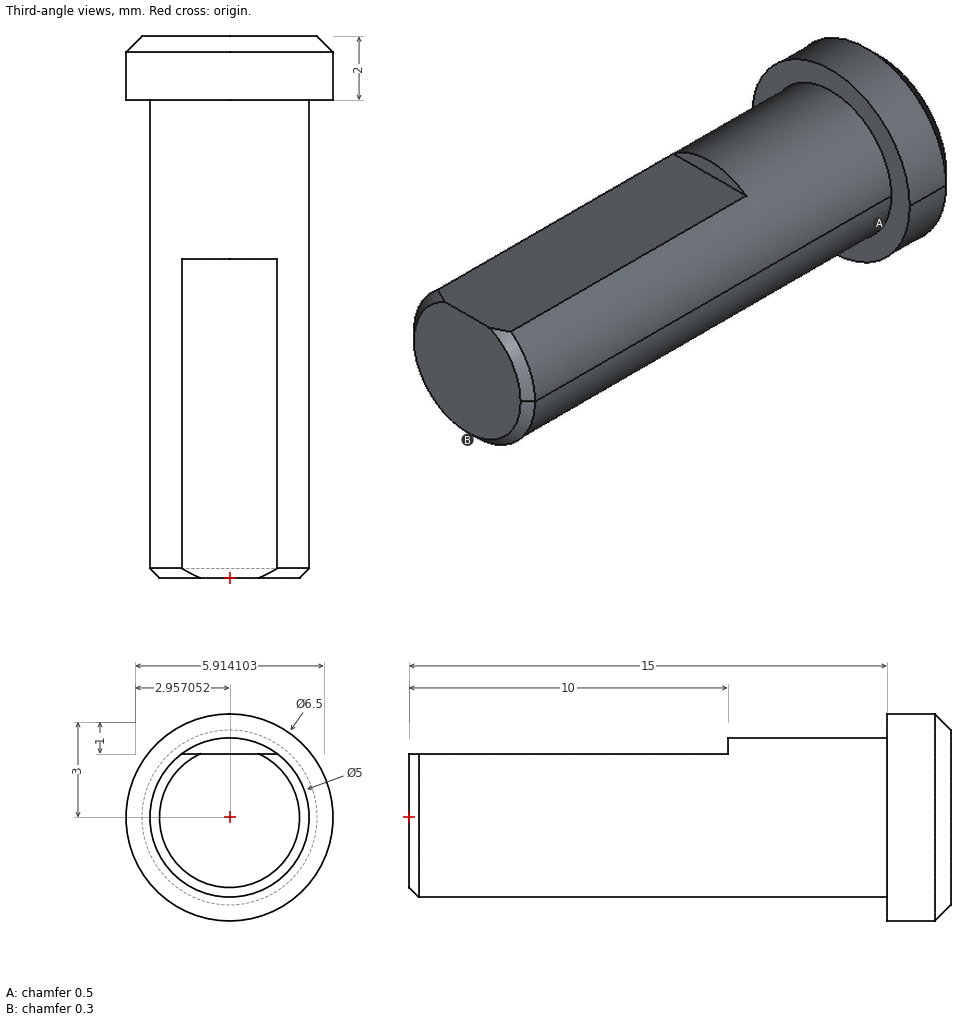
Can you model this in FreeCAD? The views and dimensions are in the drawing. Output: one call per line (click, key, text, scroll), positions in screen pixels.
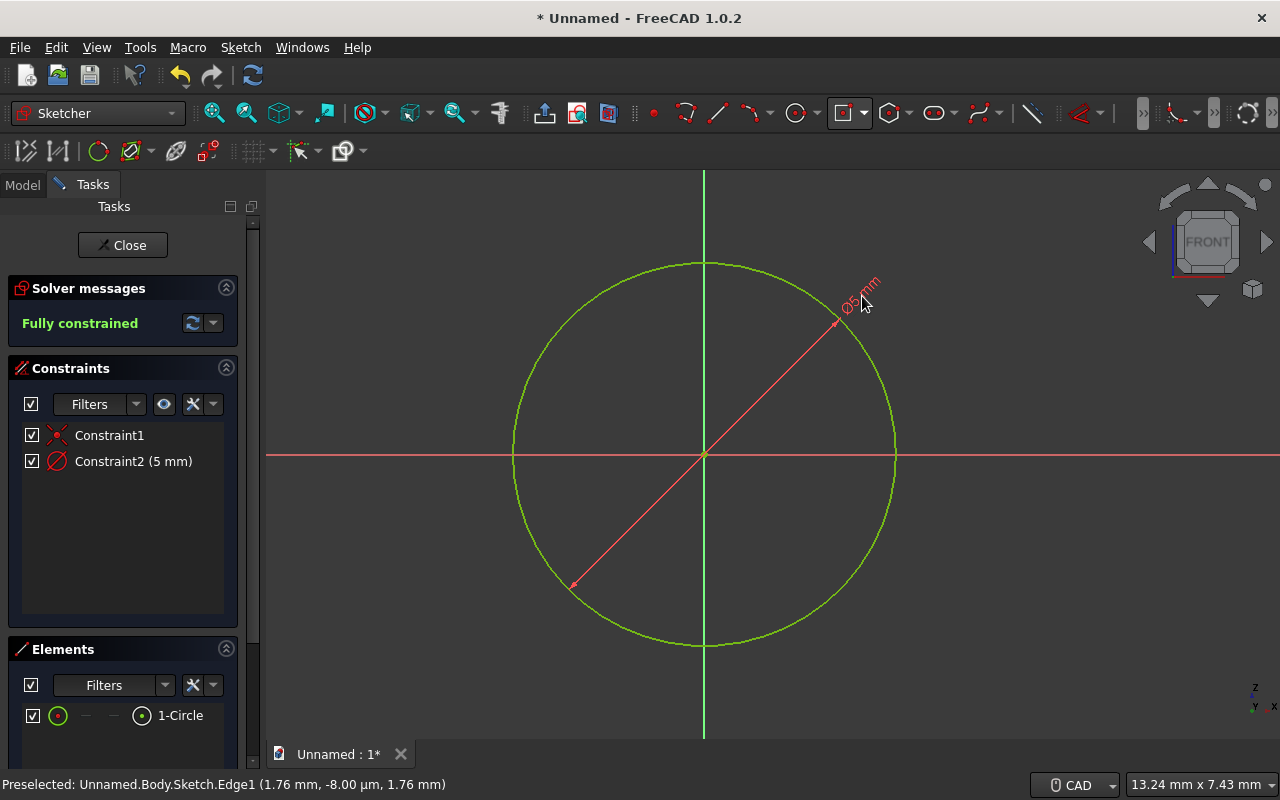
click(123, 245)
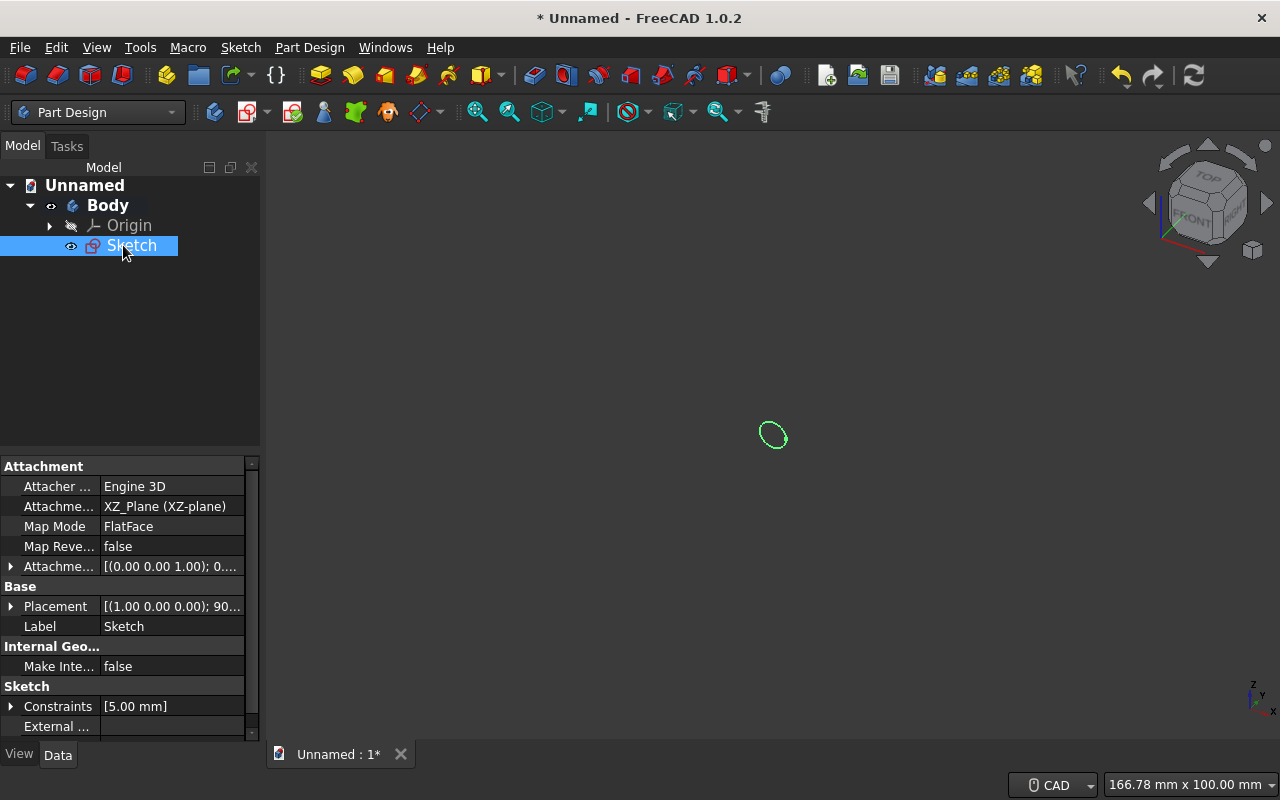
click(322, 76)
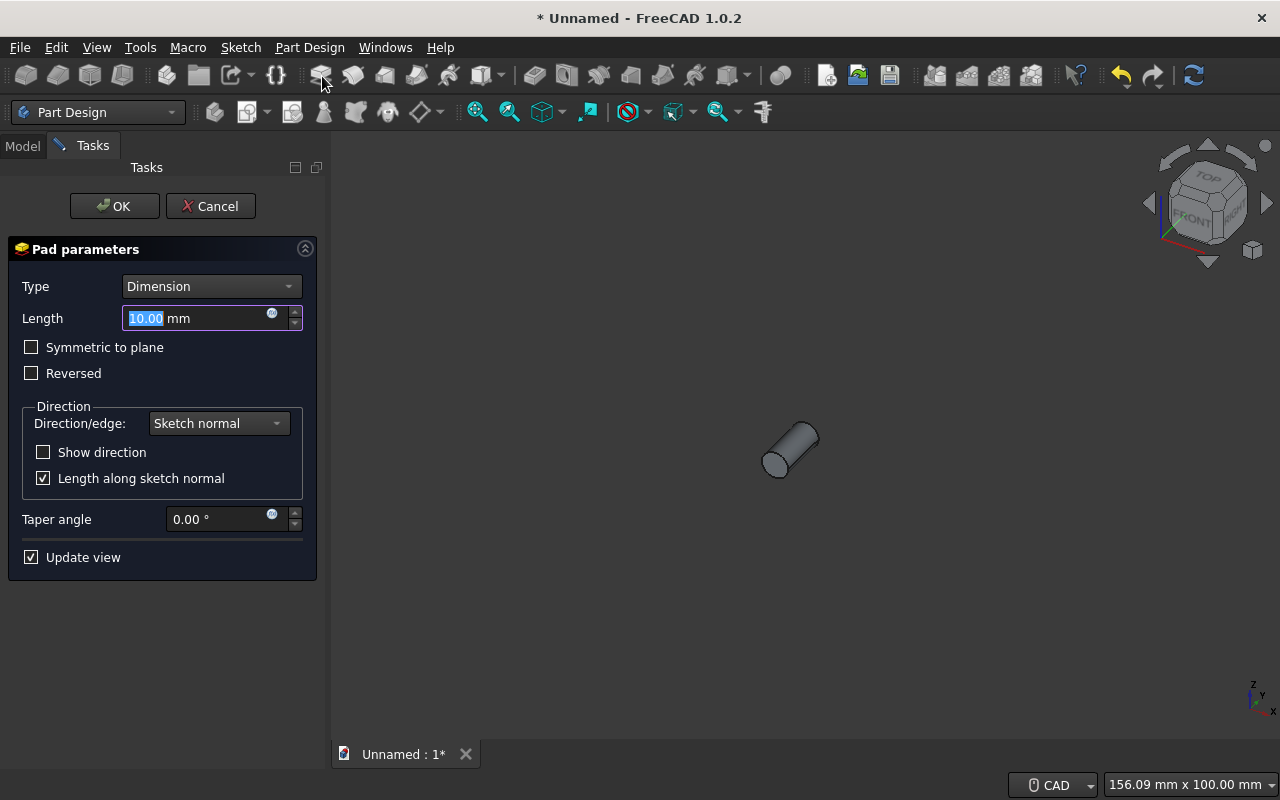
text(15)
key(Tab)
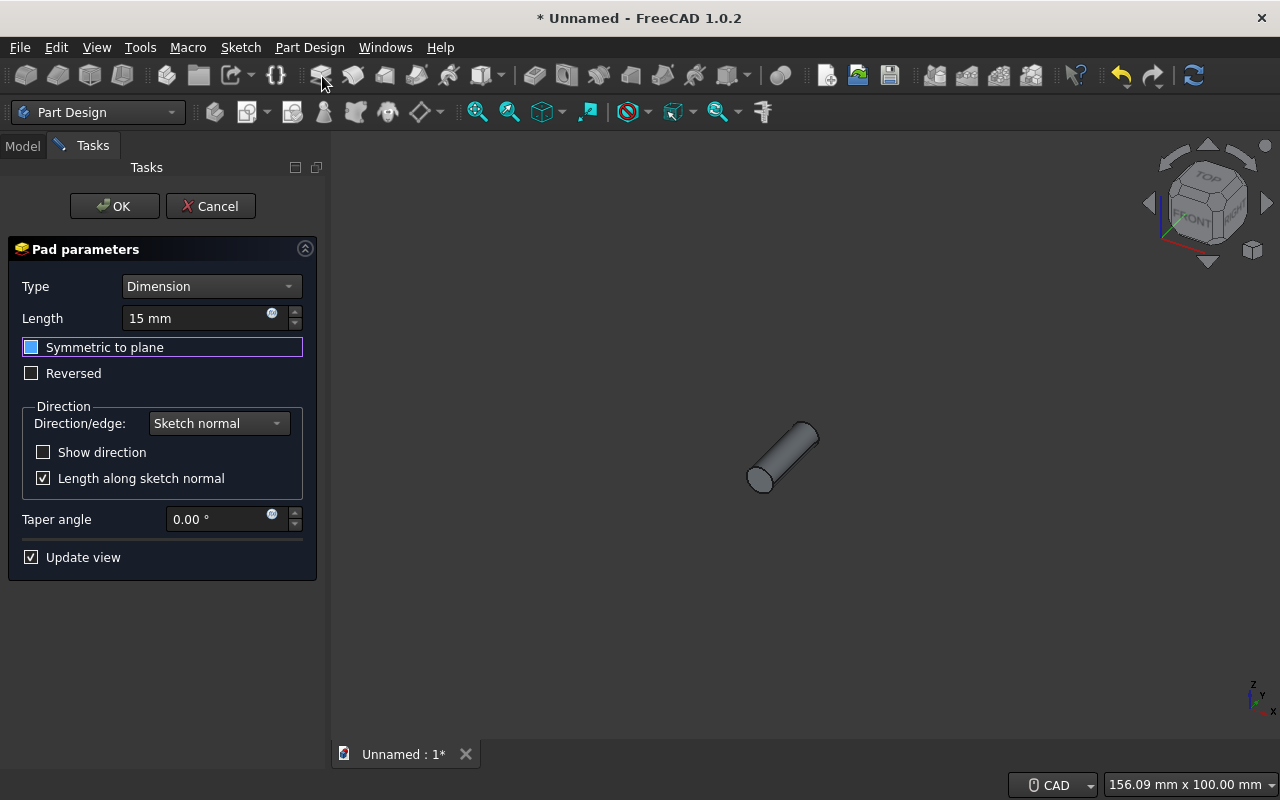
click(30, 373)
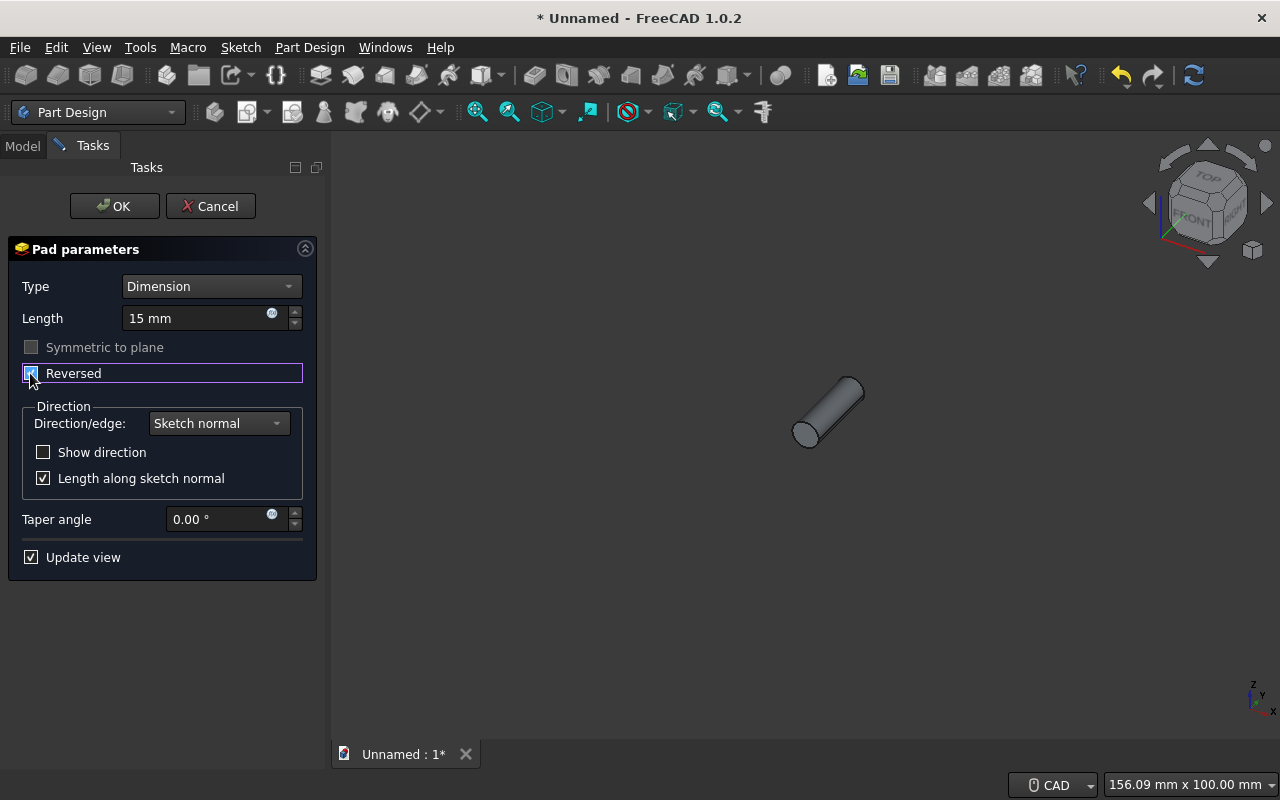
click(115, 206)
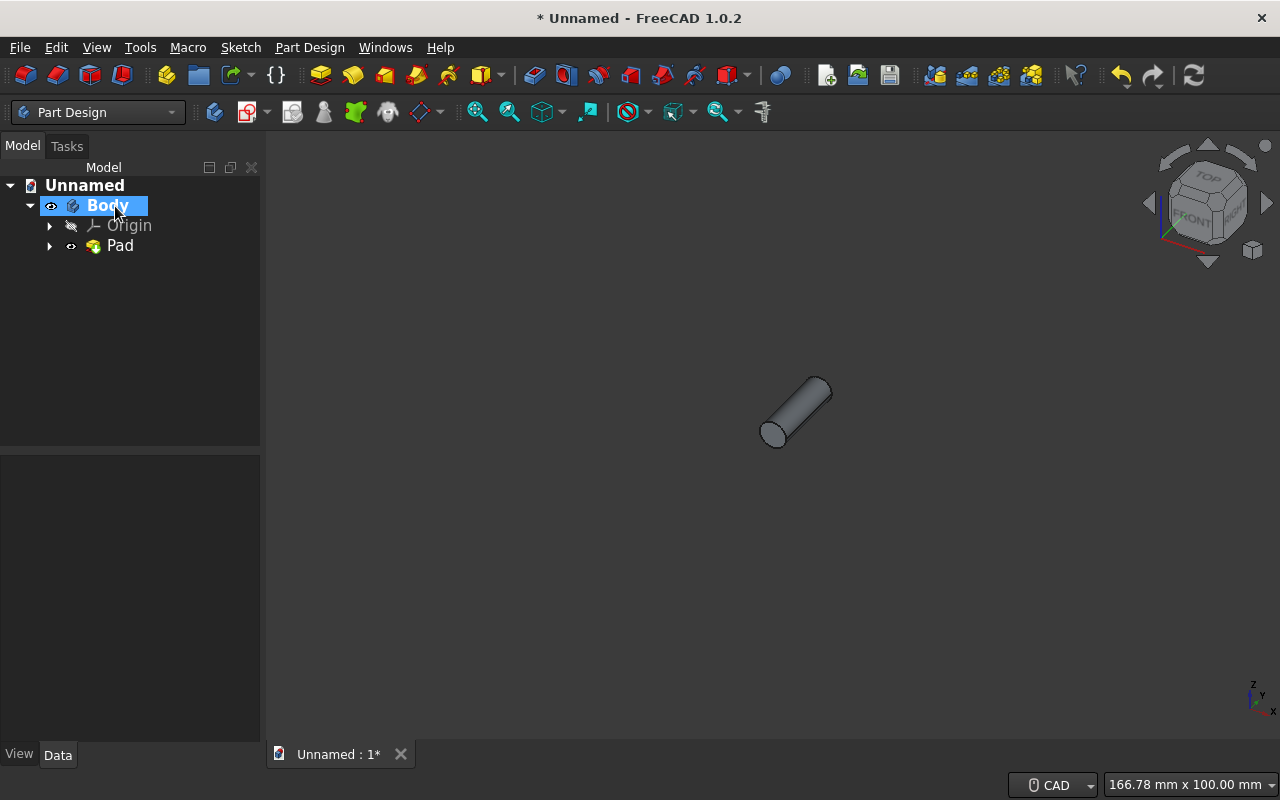
click(478, 112)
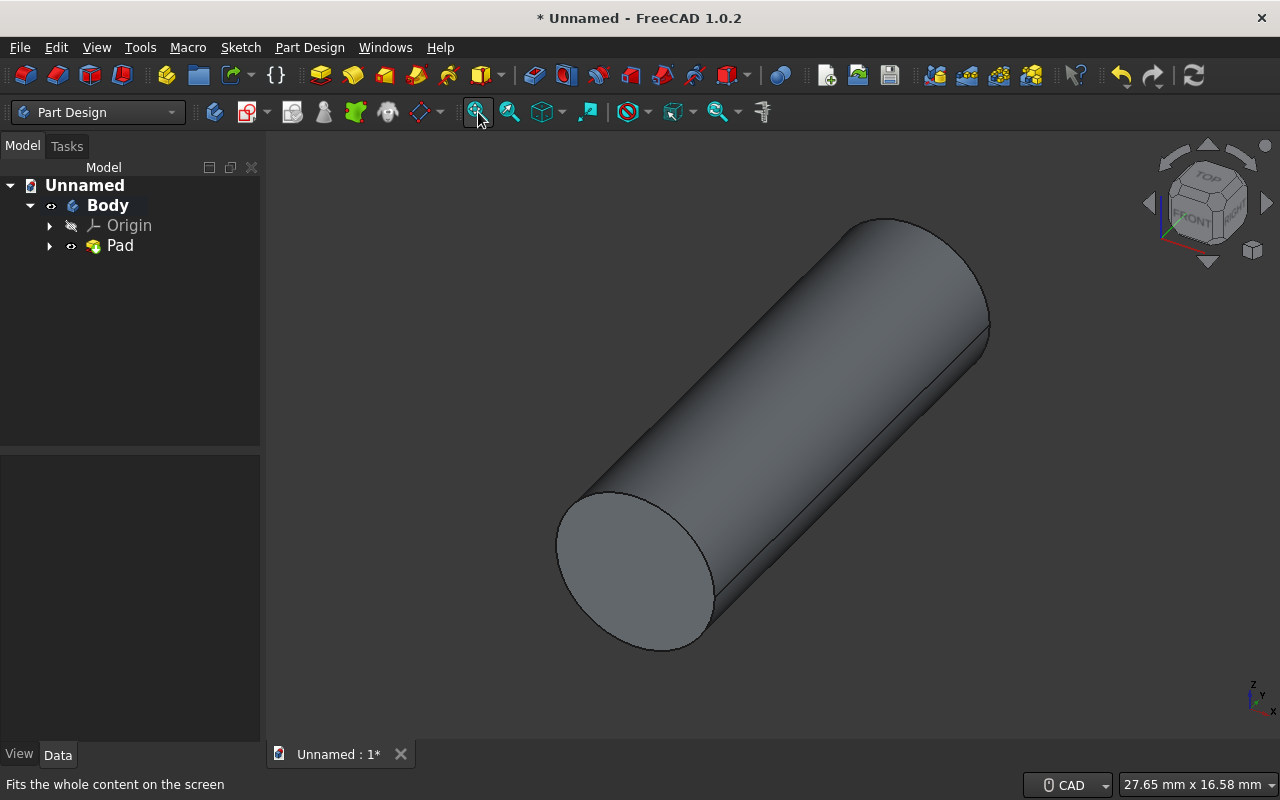
key(4)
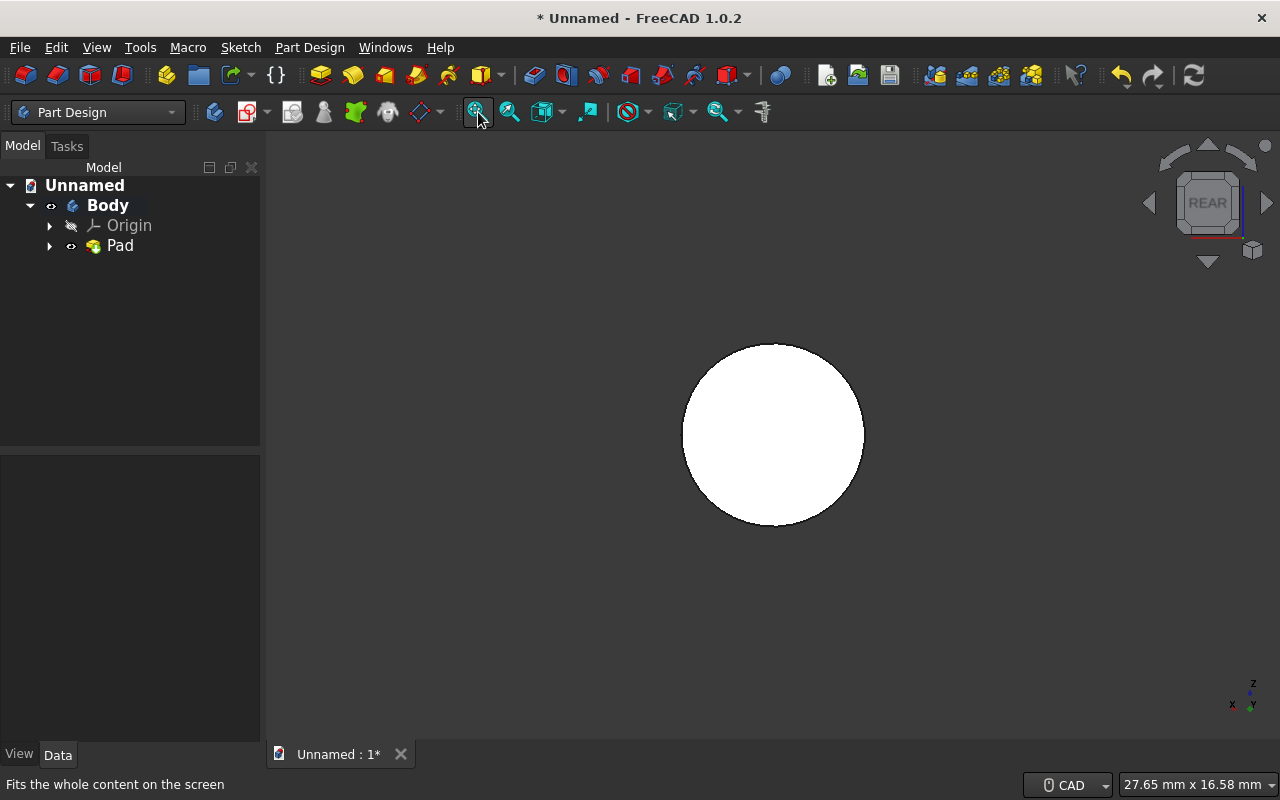
click(478, 112)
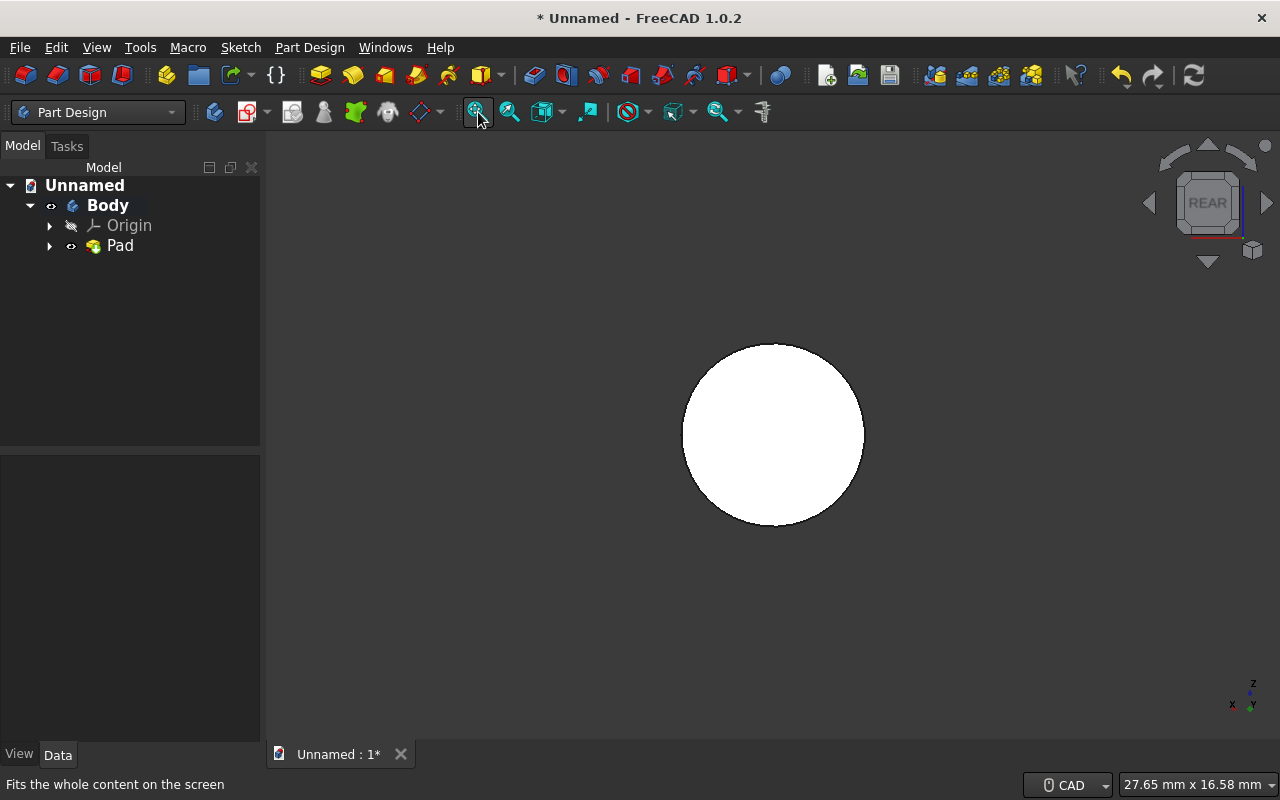
click(773, 434)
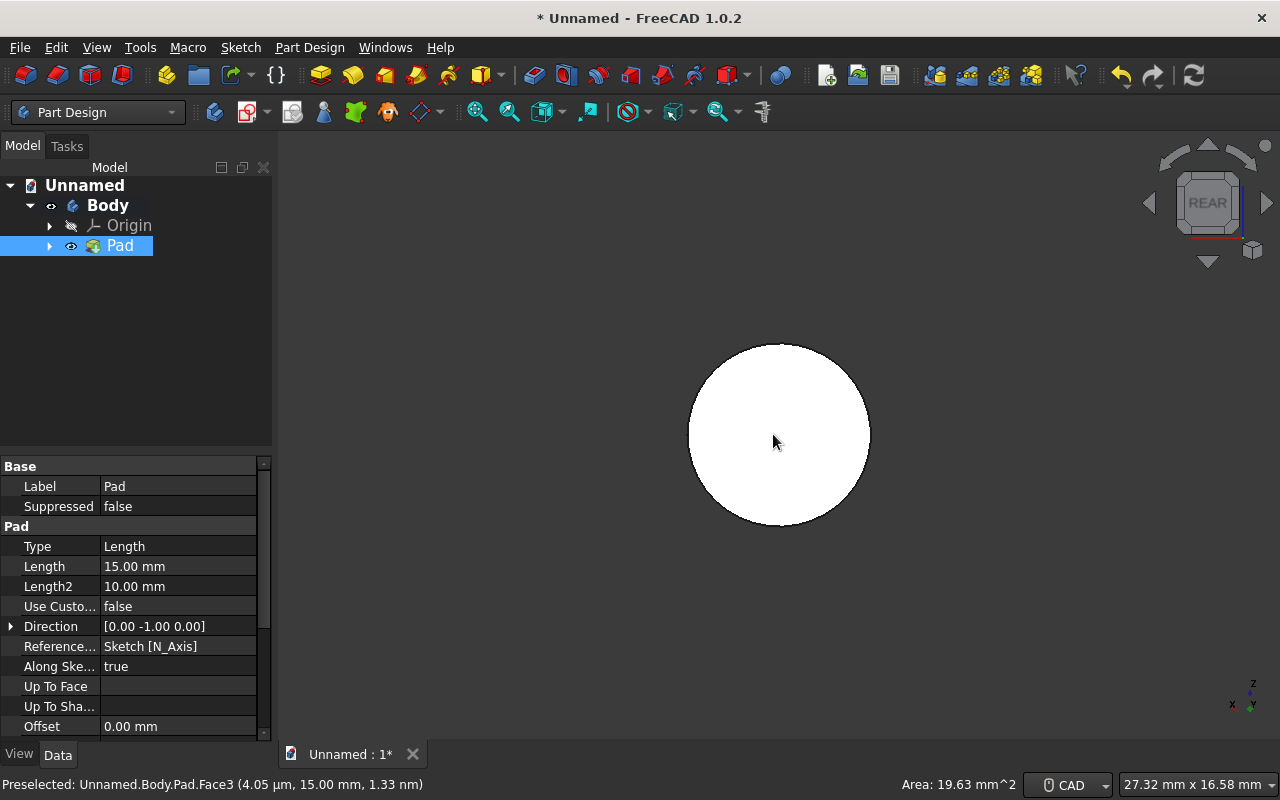
click(248, 112)